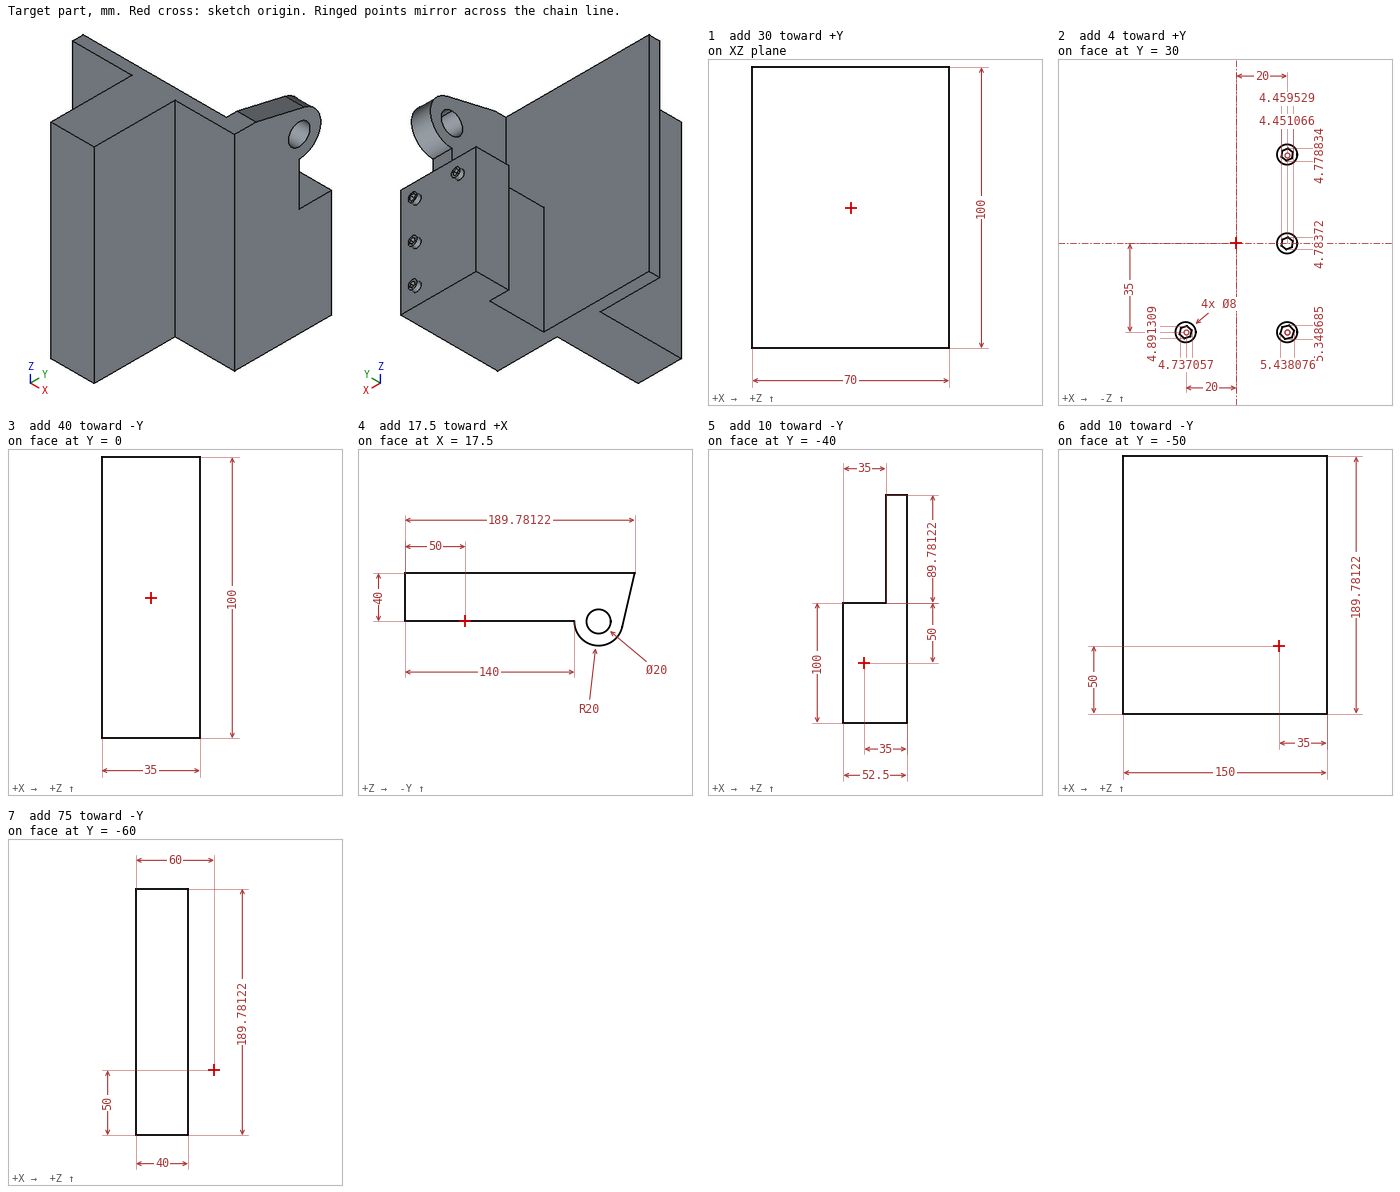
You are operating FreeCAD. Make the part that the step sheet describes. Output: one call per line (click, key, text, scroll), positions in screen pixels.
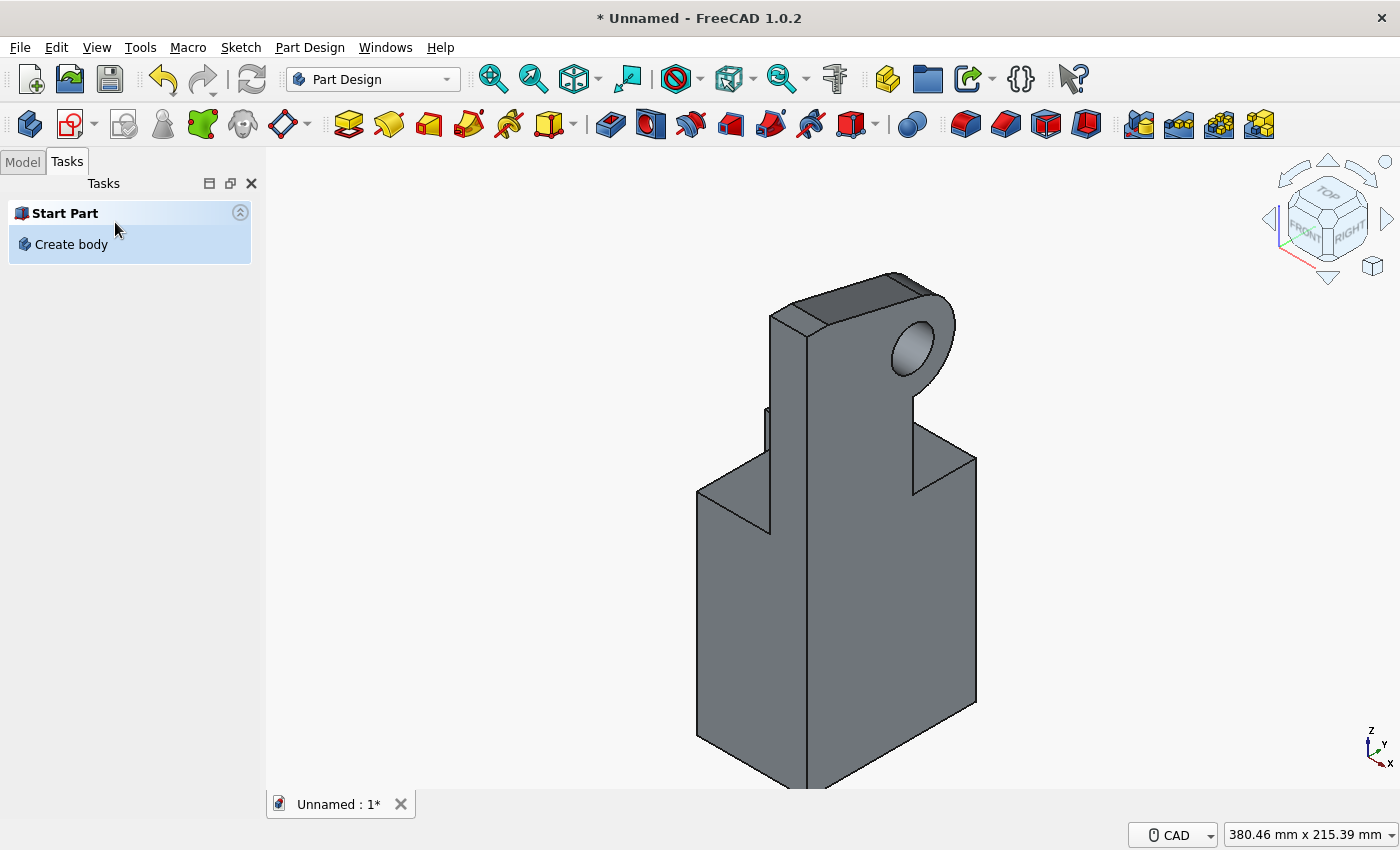
click(494, 80)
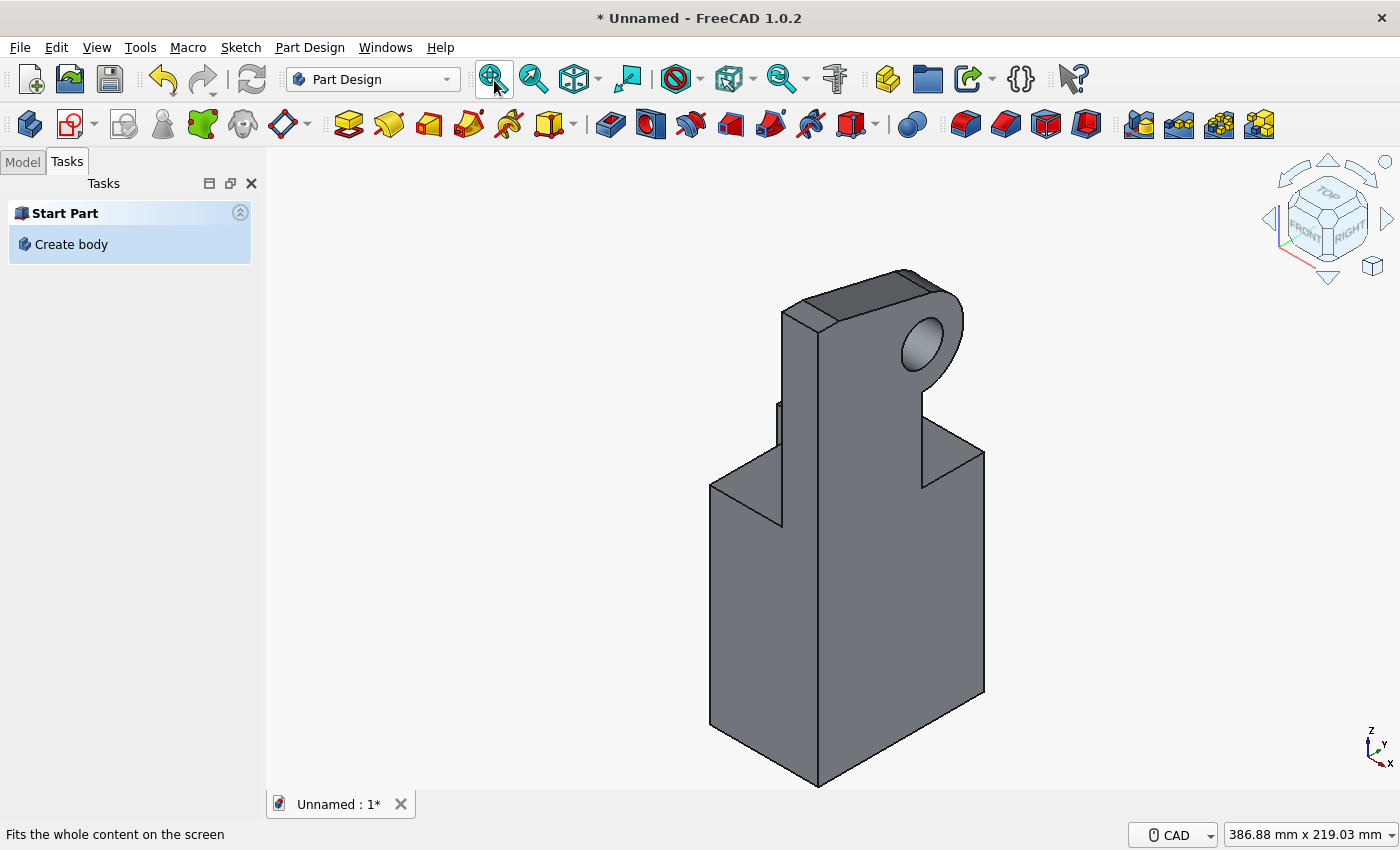
click(764, 593)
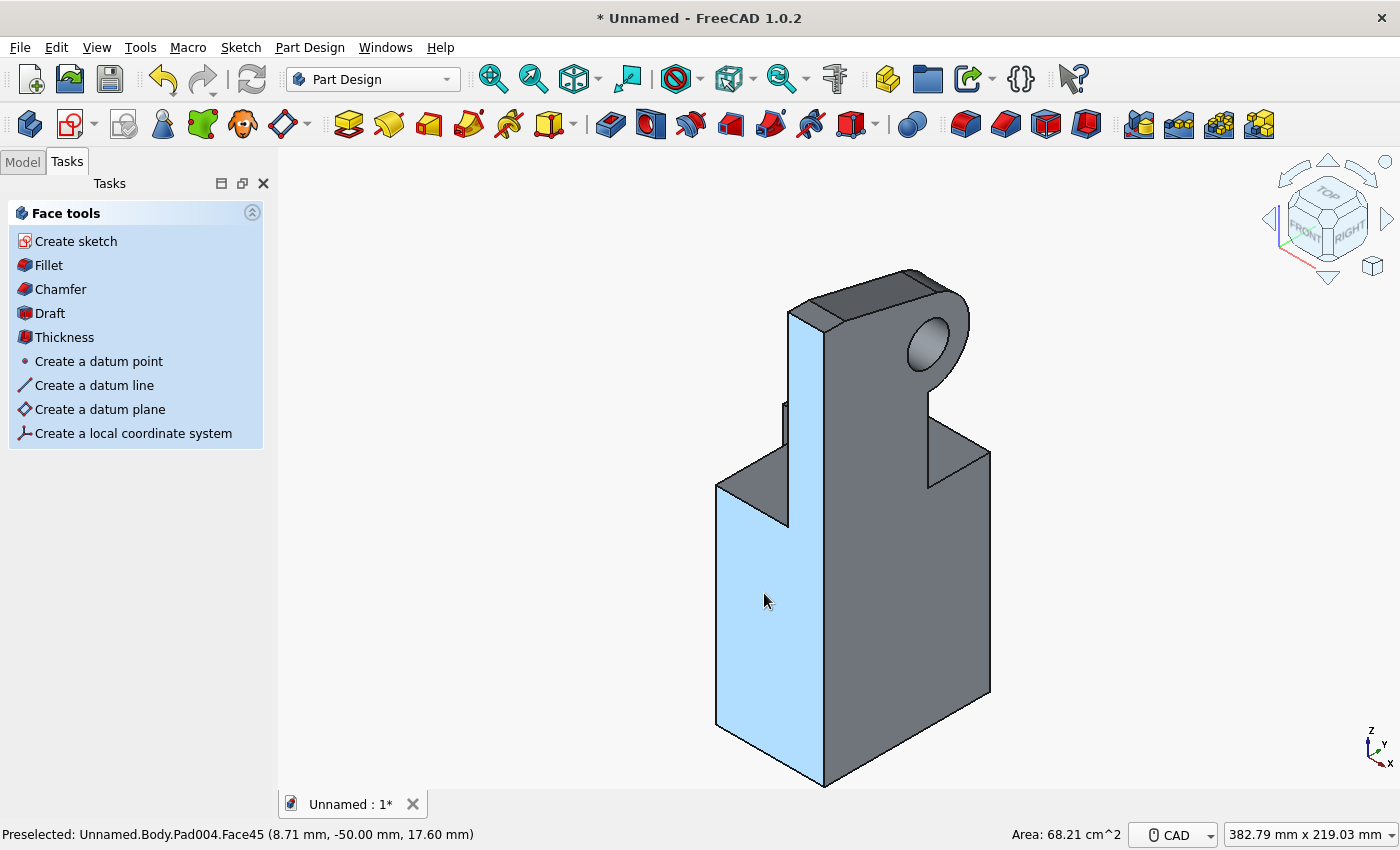
click(70, 124)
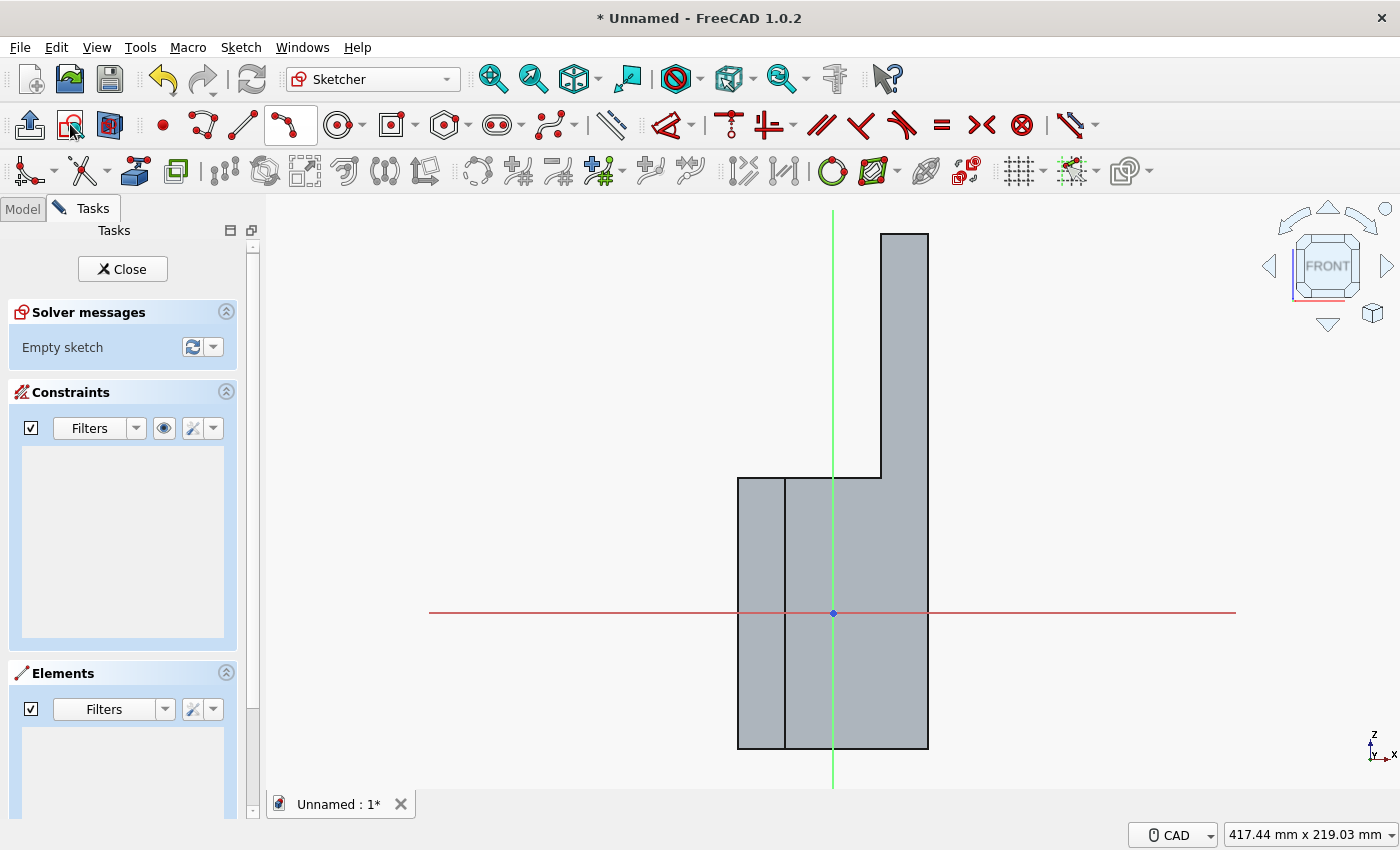
scroll(846, 491, down, 2)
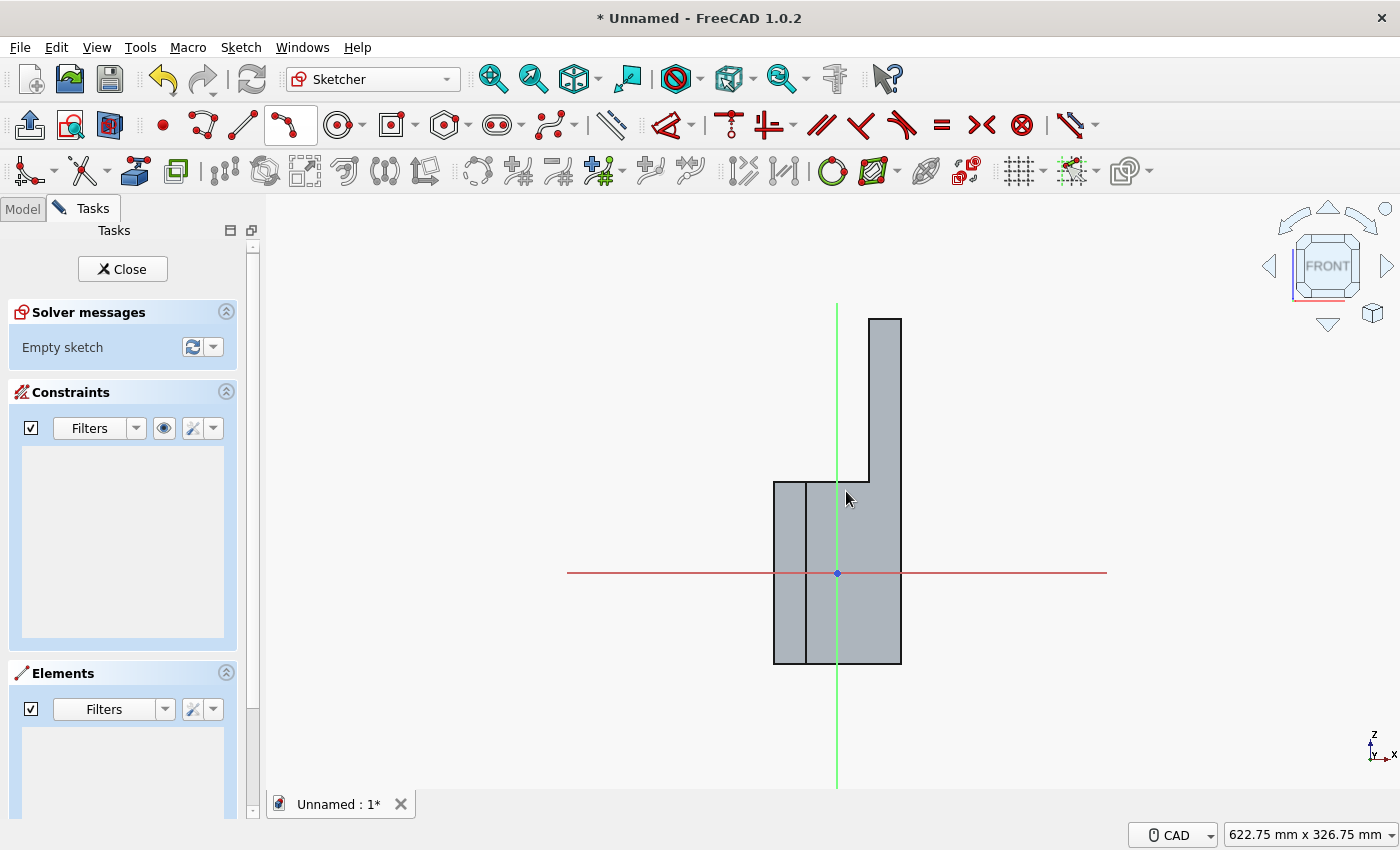
click(418, 126)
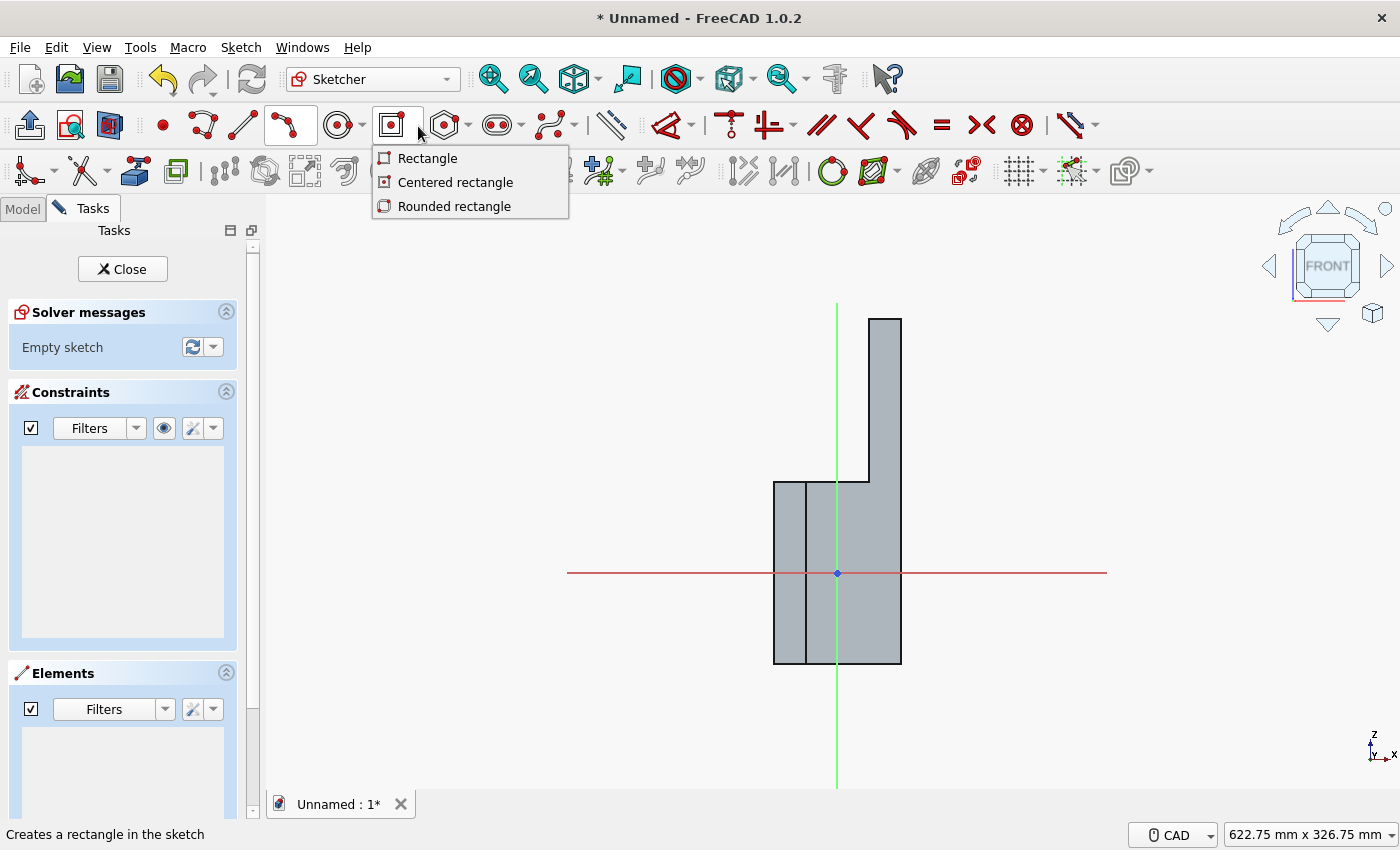
click(470, 158)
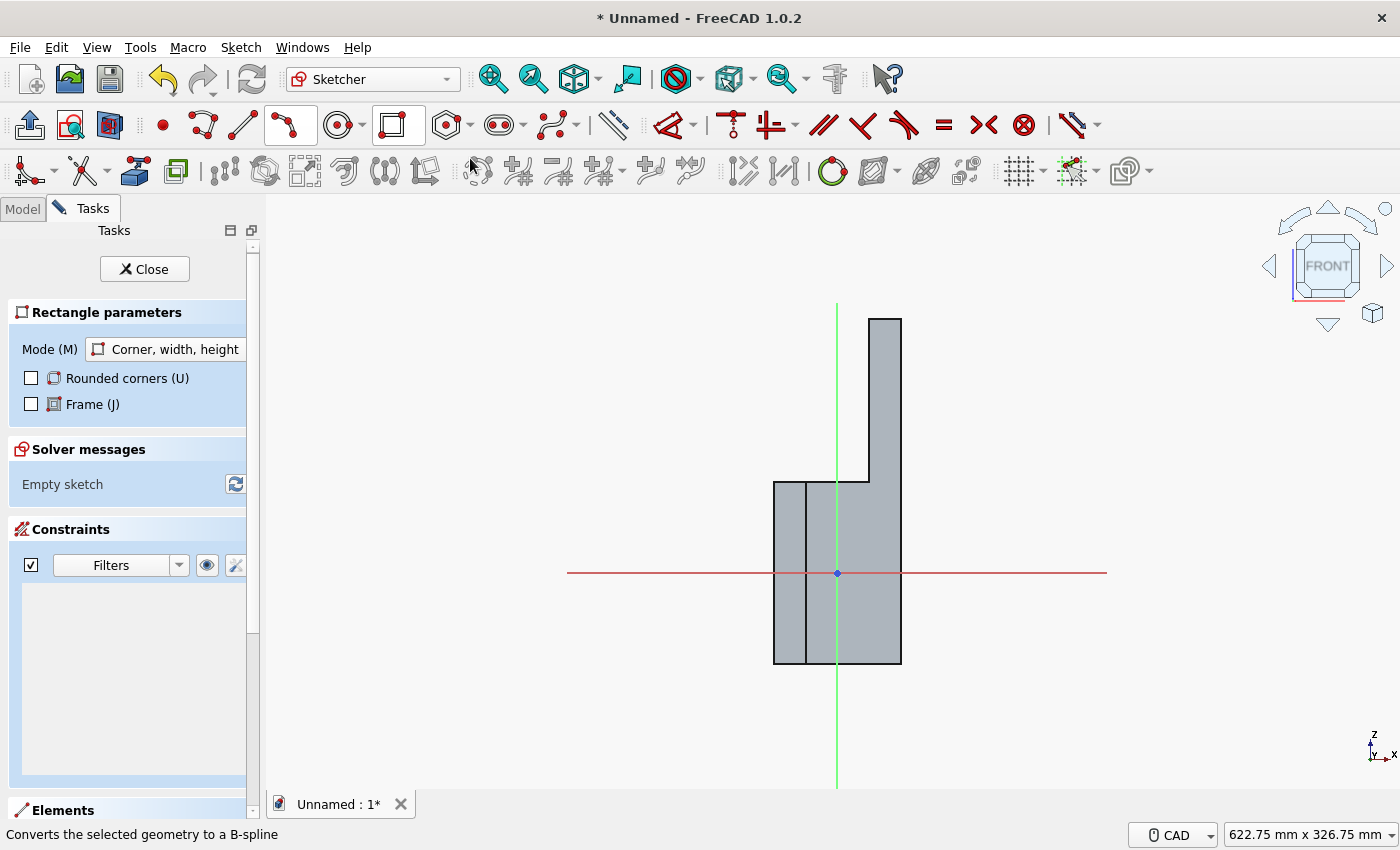
click(628, 319)
move(901, 664)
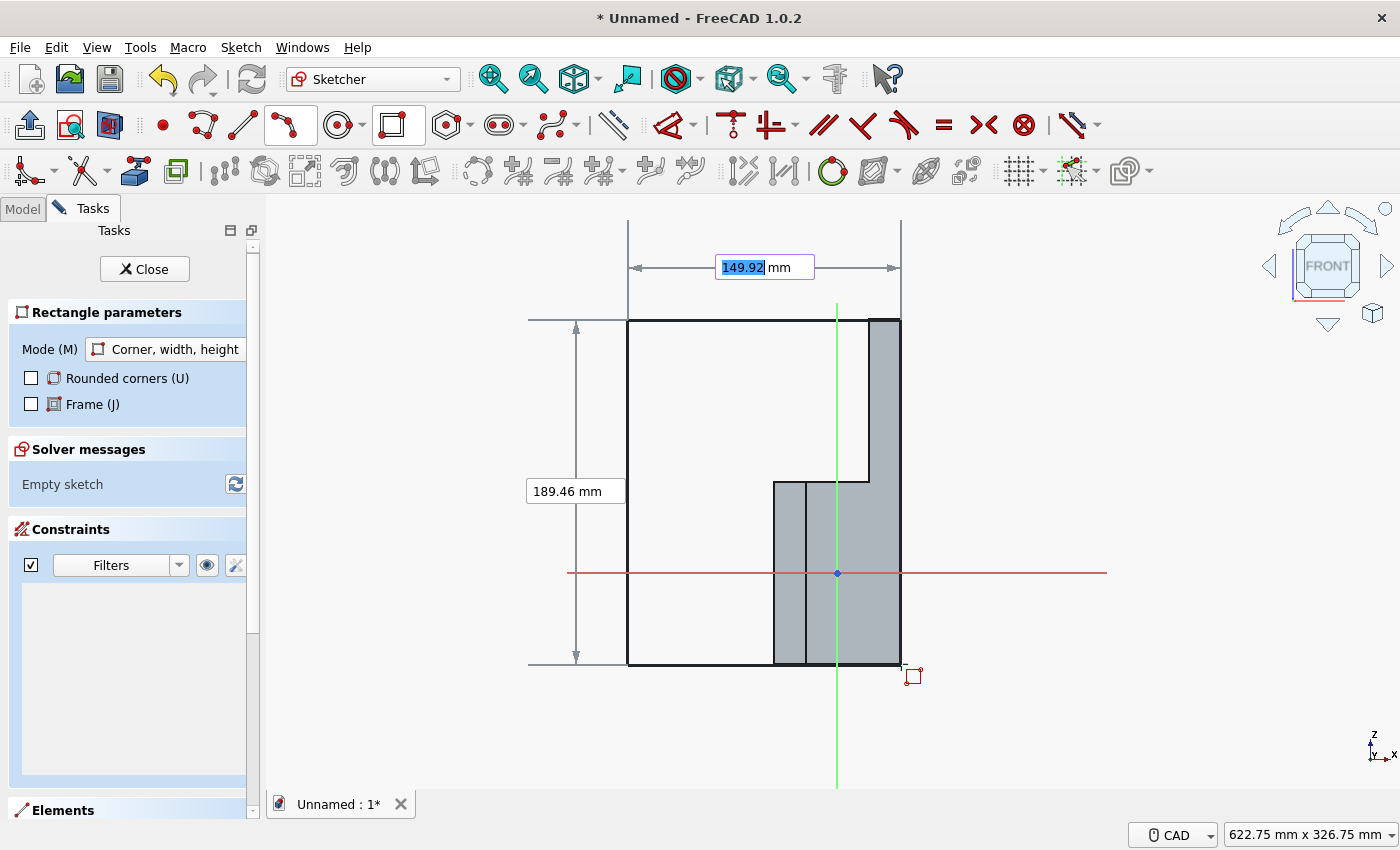
text(150)
key(Tab)
text(189.78122)
key(Return)
key(Escape)